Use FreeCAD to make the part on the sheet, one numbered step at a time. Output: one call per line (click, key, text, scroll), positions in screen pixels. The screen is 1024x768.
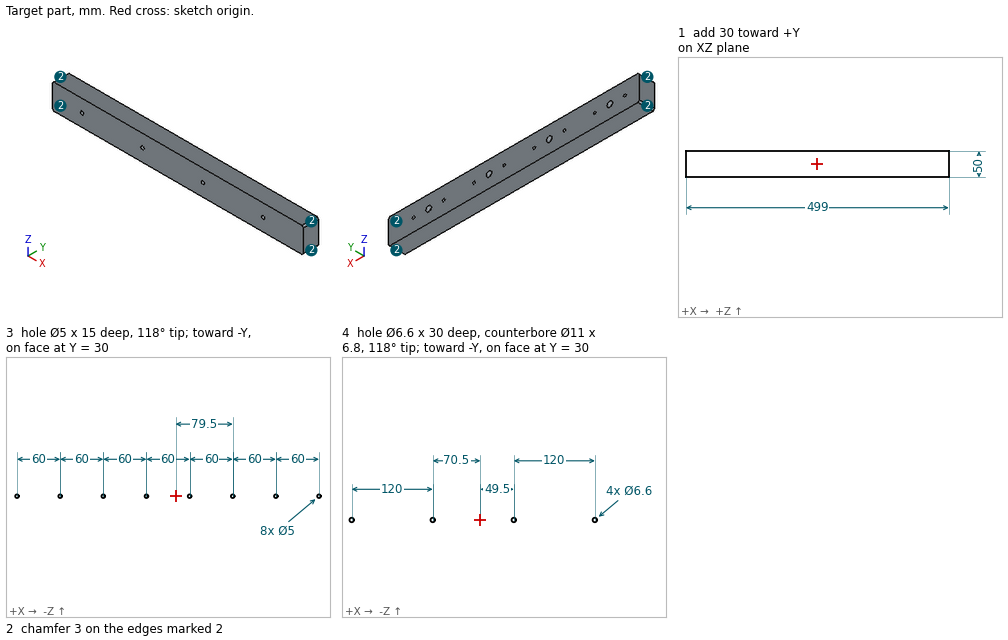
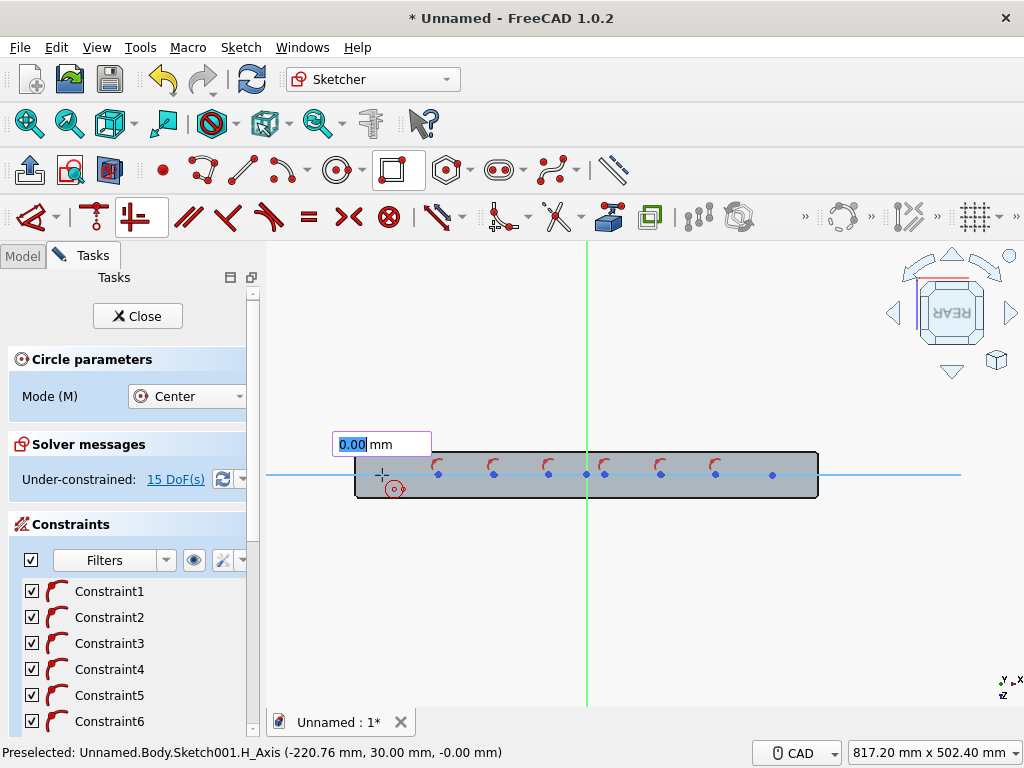
scroll(381, 477, up, 10)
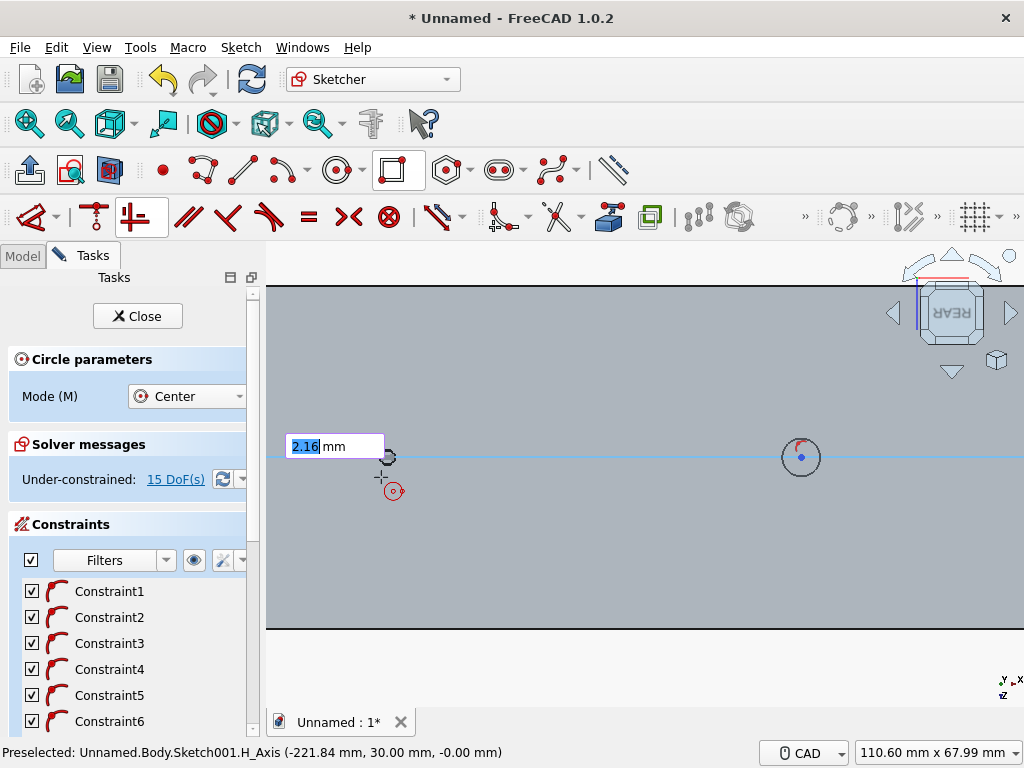
click(383, 474)
key(Escape)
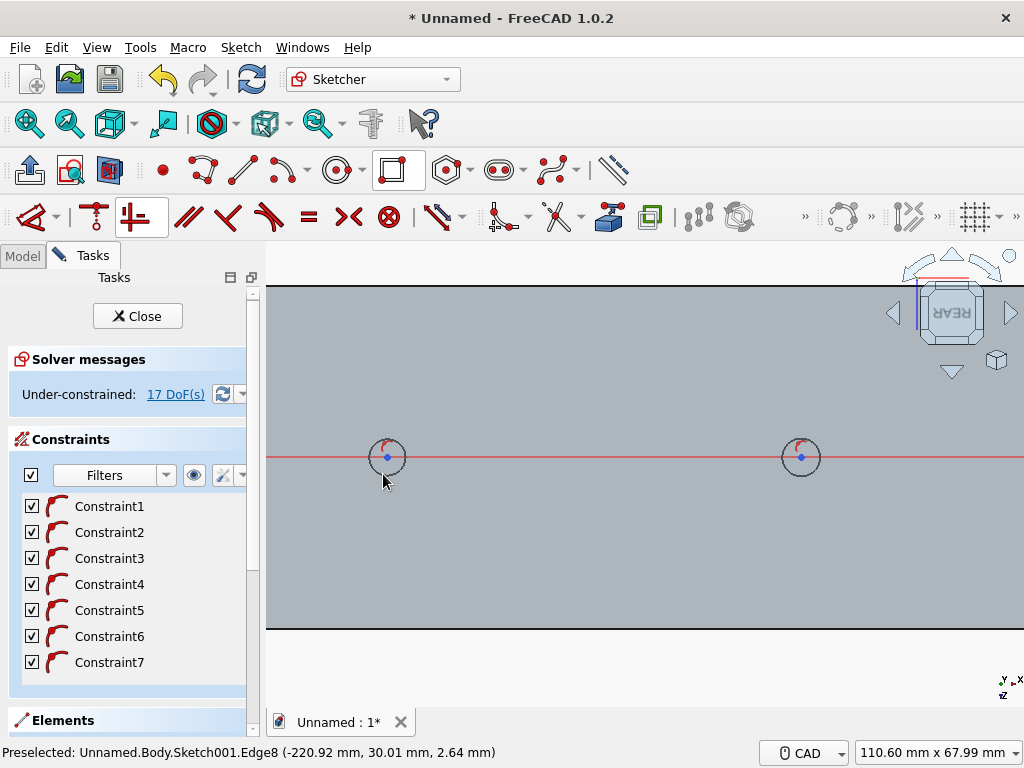
scroll(381, 477, down, 10)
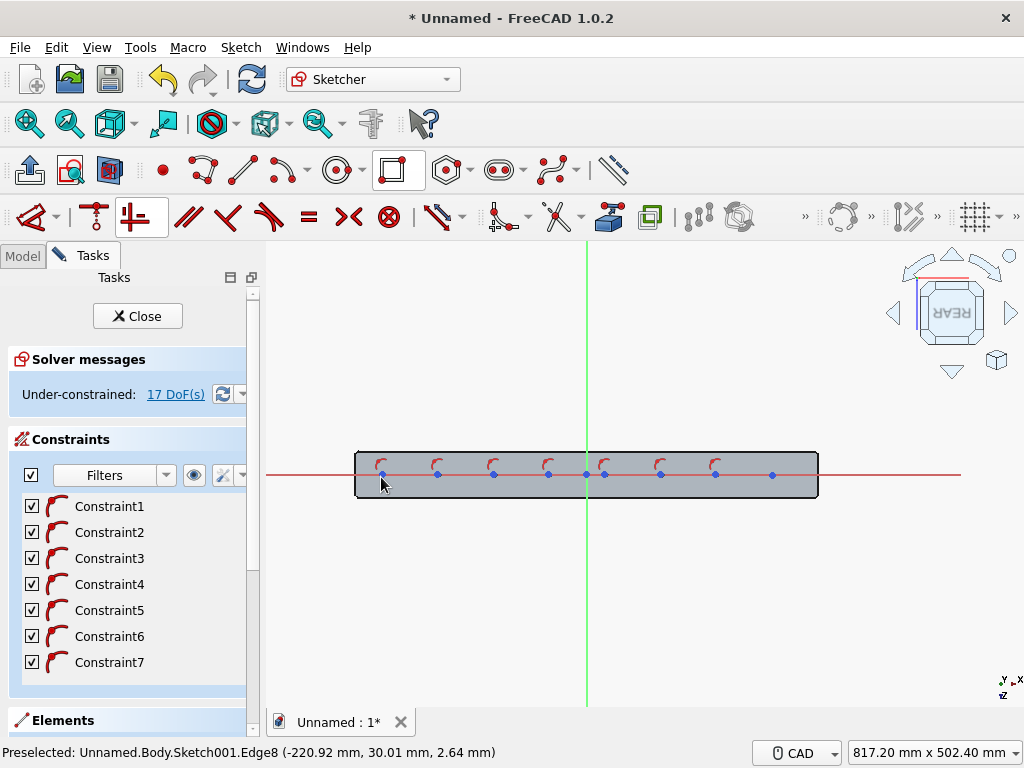
scroll(773, 475, up, 12)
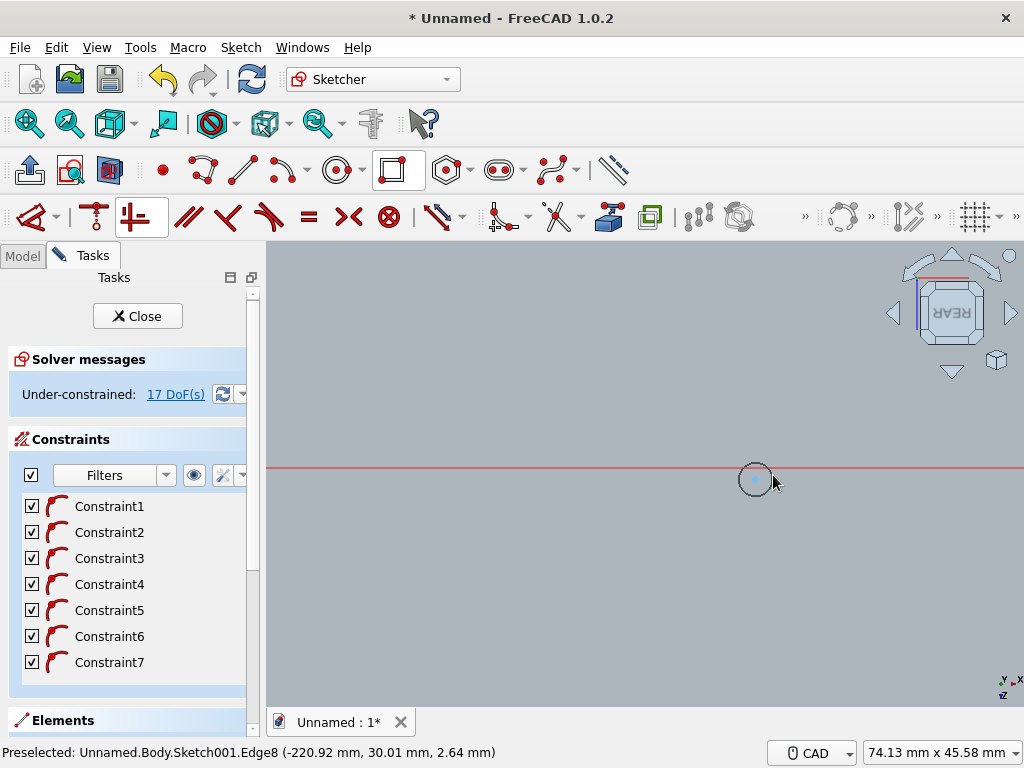
click(767, 468)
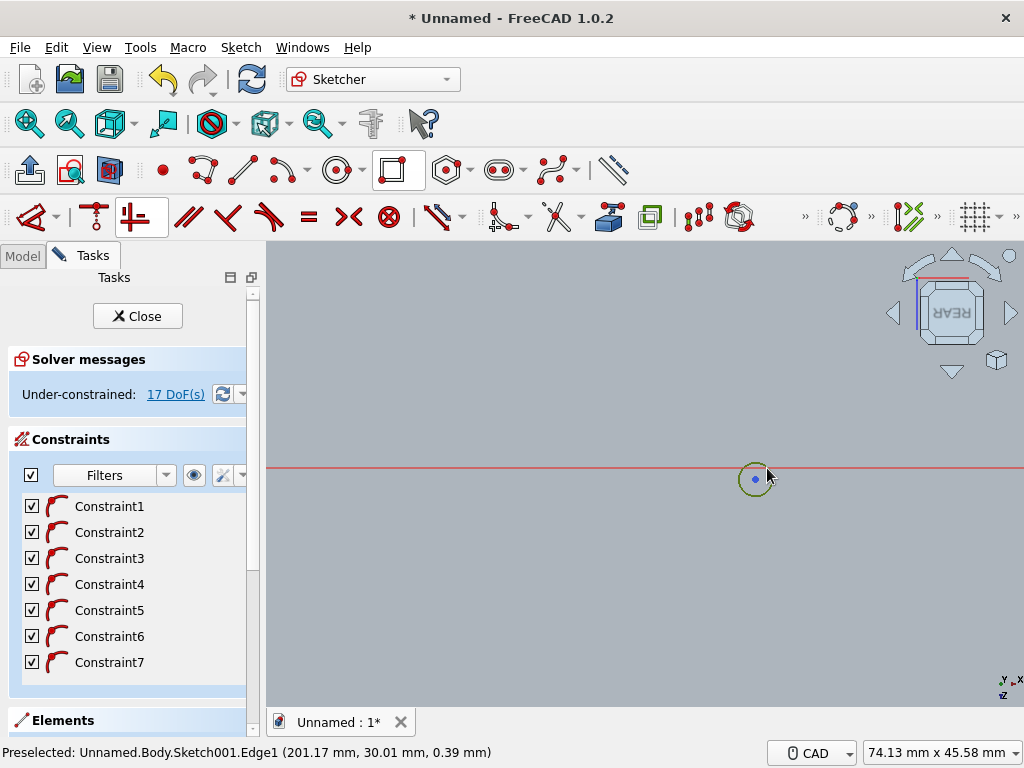
scroll(773, 475, down, 12)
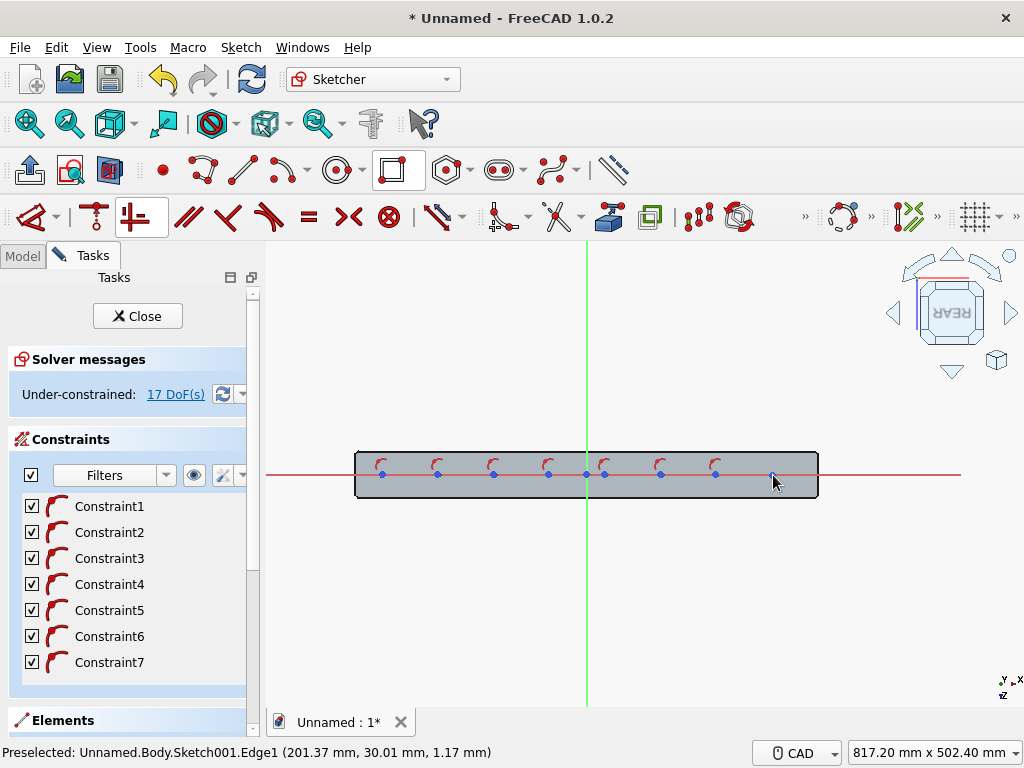
scroll(718, 473, up, 11)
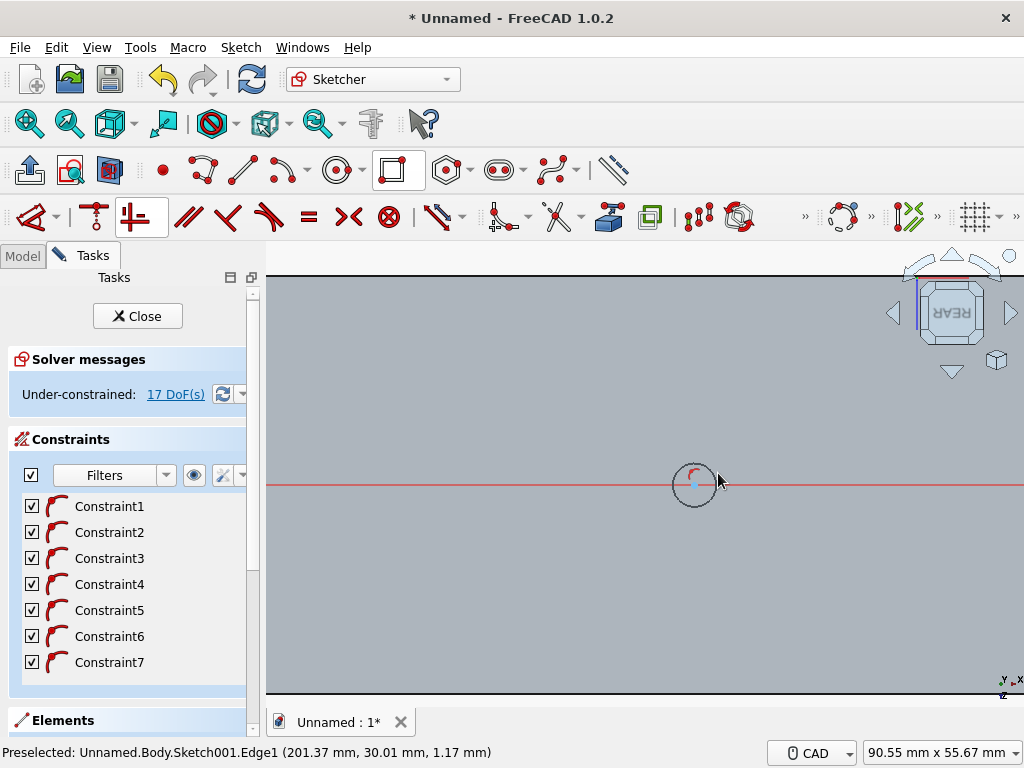
click(710, 470)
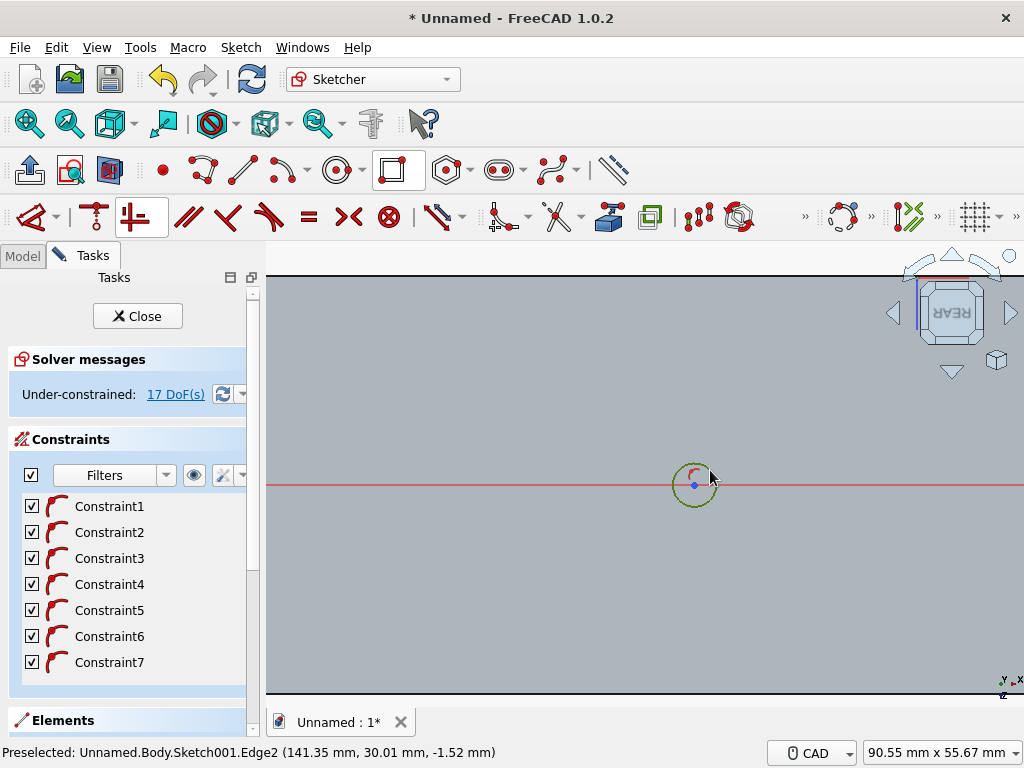
scroll(718, 473, down, 11)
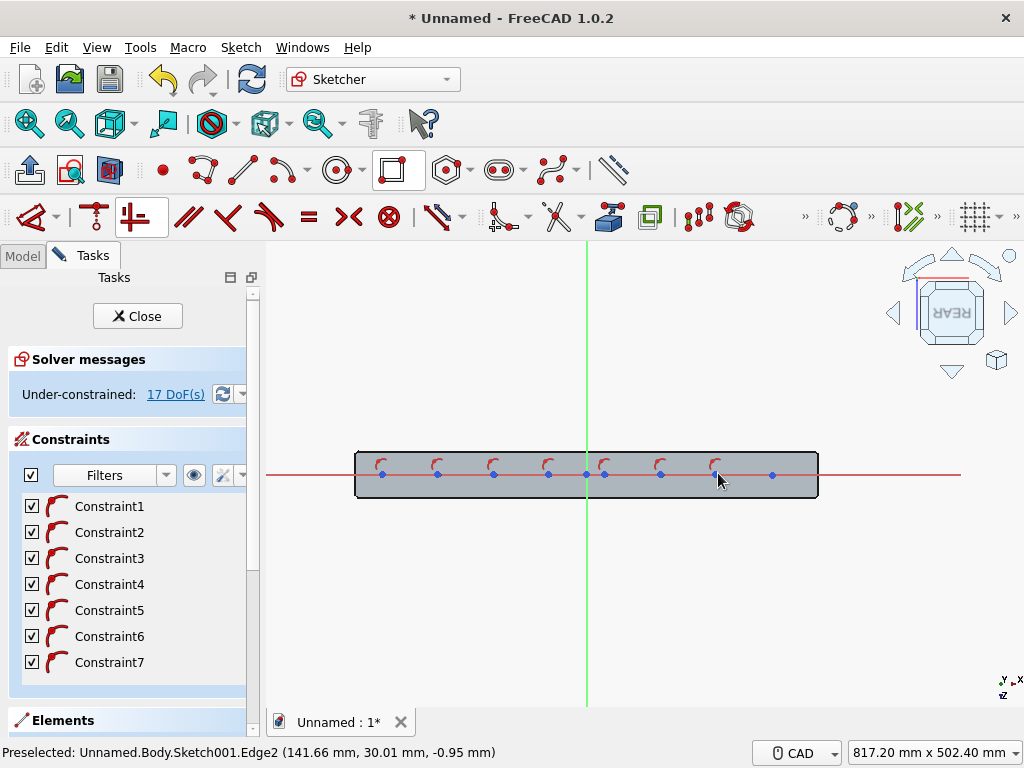
scroll(663, 473, up, 10)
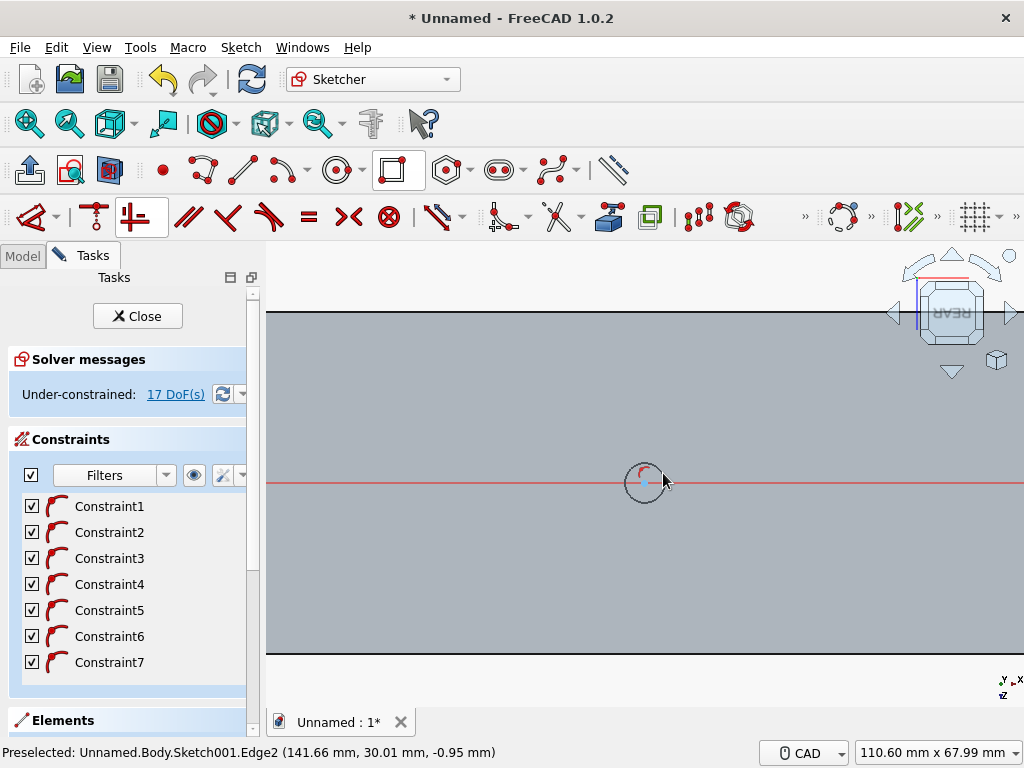
click(659, 469)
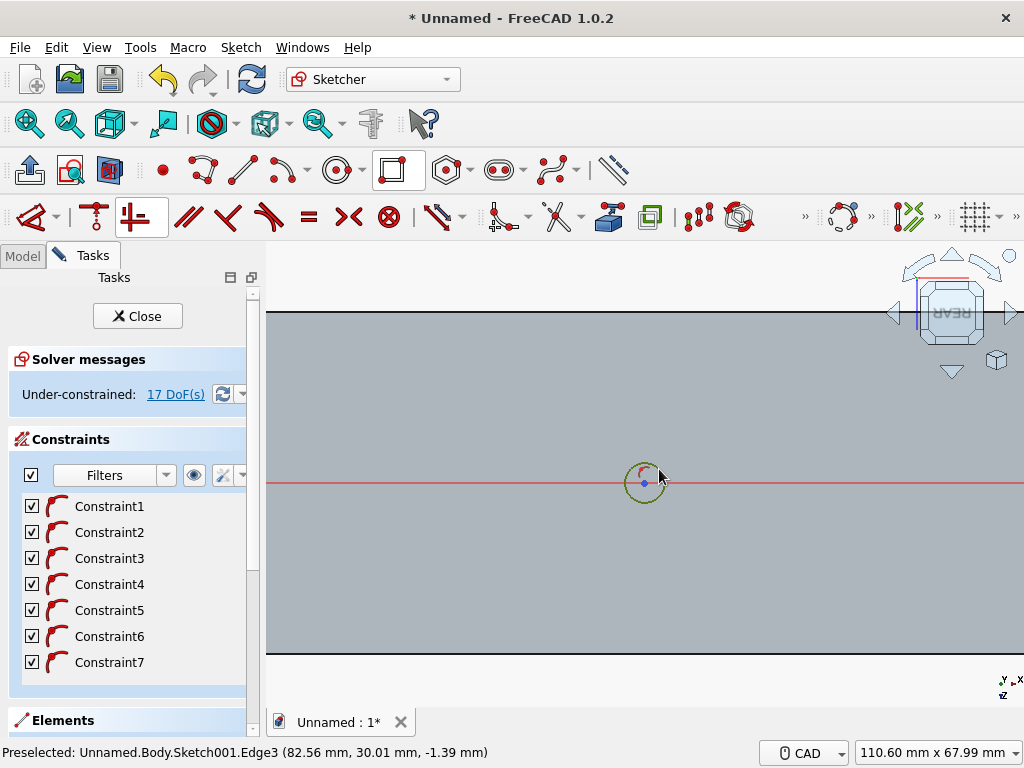
scroll(663, 473, down, 10)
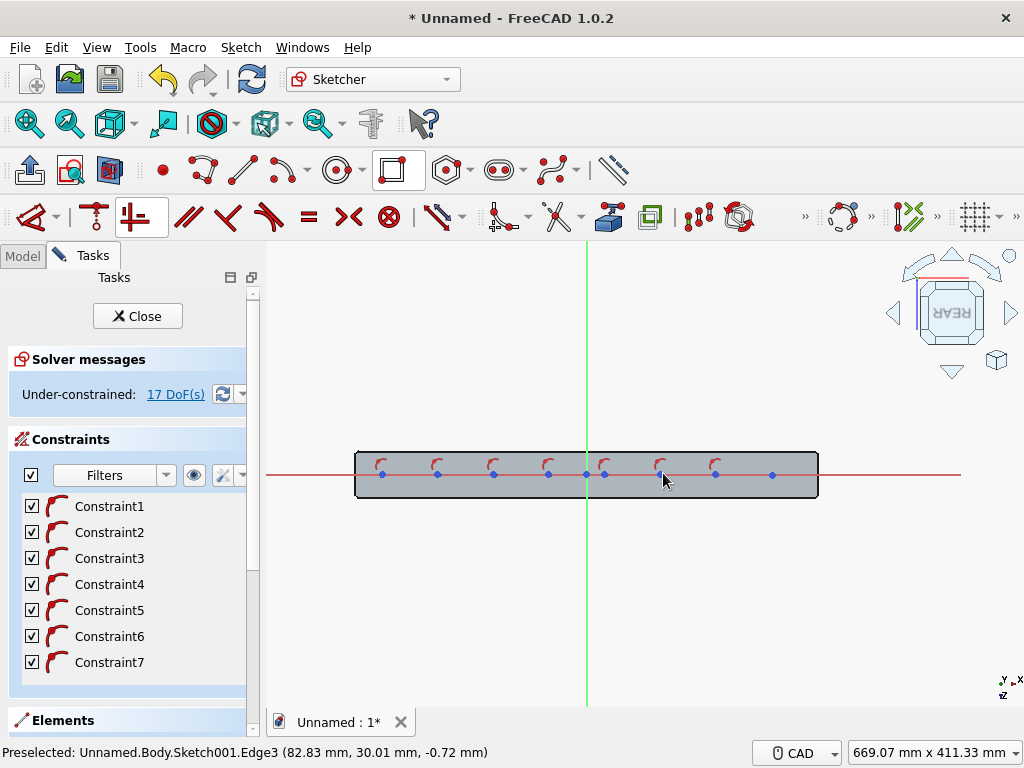
scroll(607, 473, up, 11)